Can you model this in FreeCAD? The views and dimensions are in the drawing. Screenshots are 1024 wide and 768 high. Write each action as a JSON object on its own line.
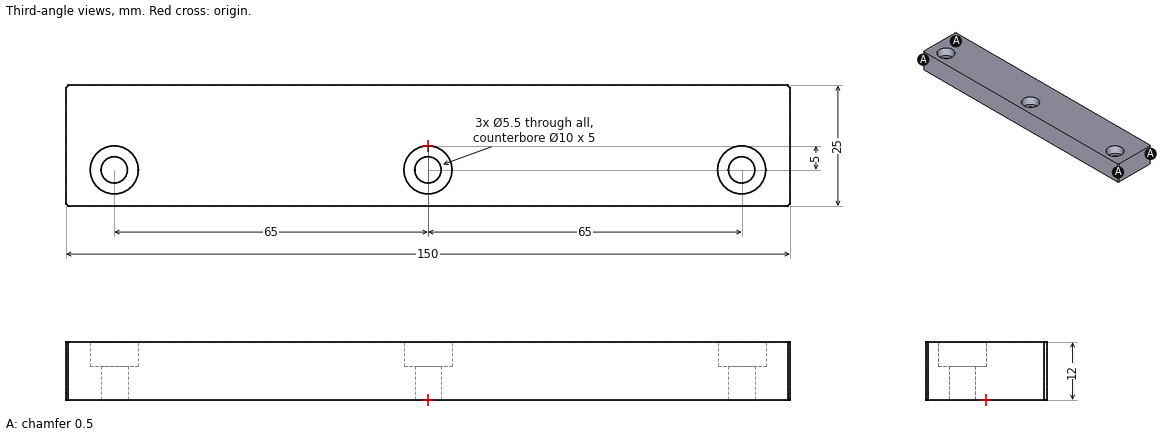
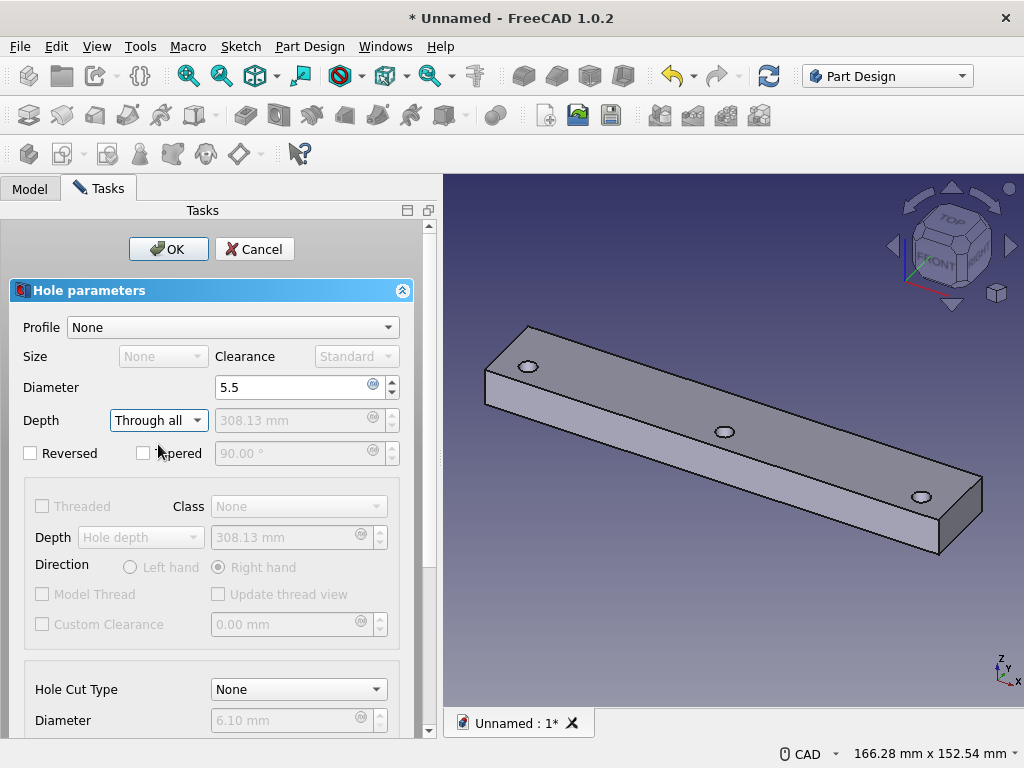
{"action": "left_click", "coordinate": [300, 690]}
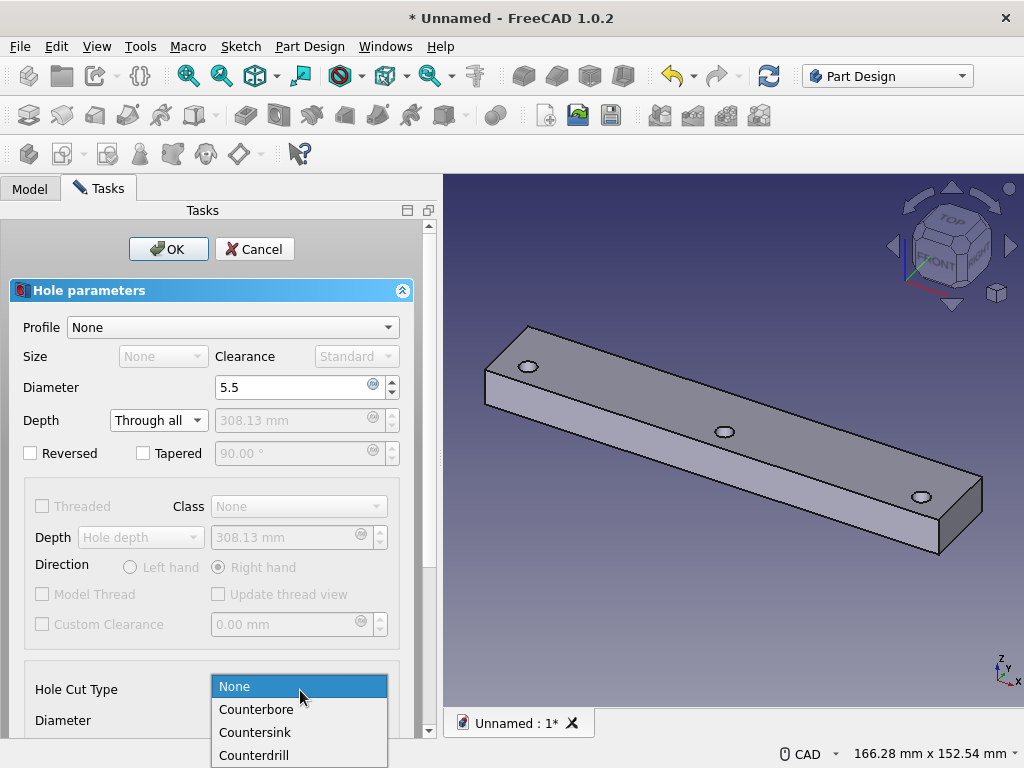
{"action": "left_click", "coordinate": [298, 710]}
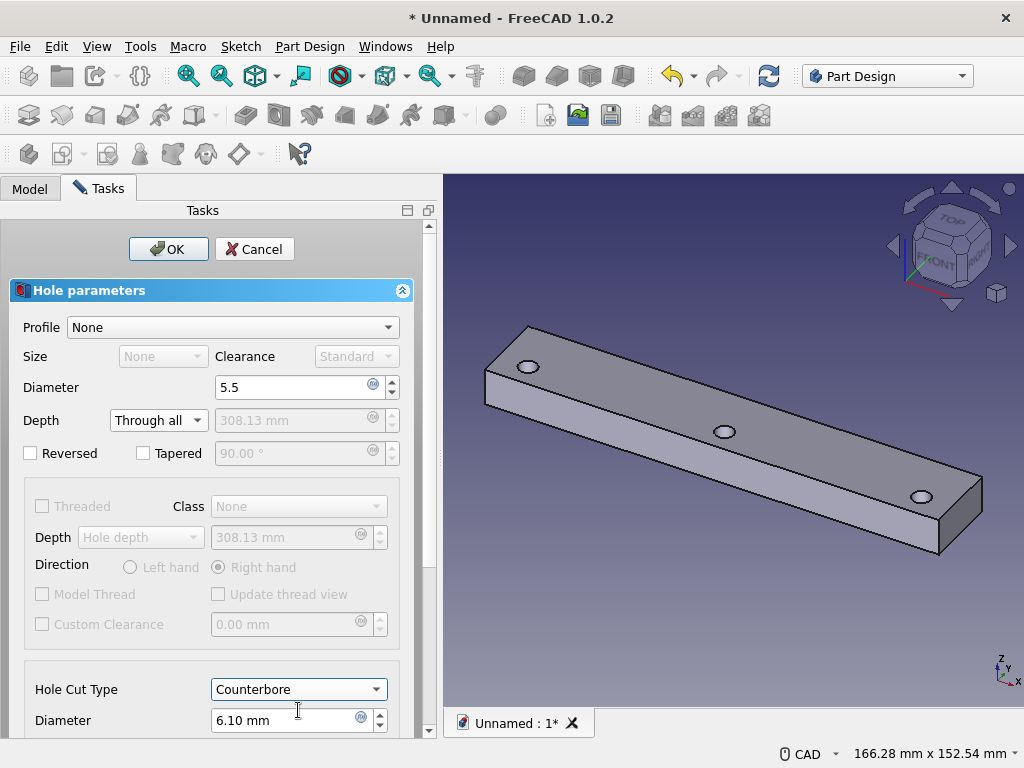
{"action": "triple_click", "coordinate": [292, 720]}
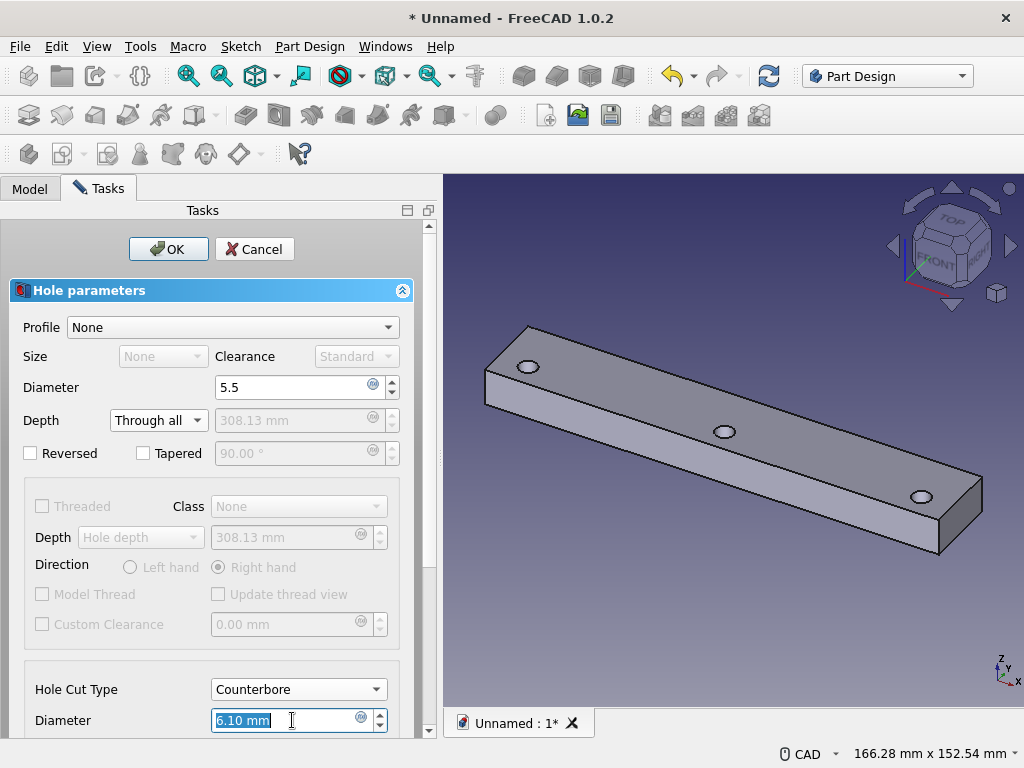
{"action": "type", "text": "10"}
{"action": "key", "text": "Tab"}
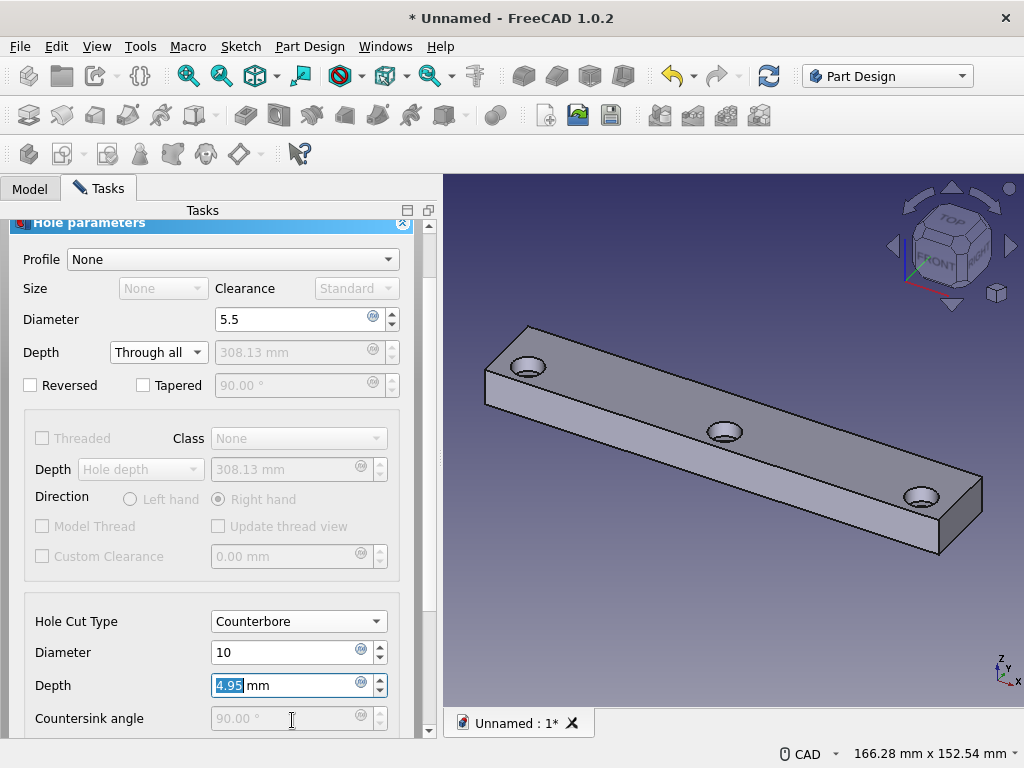
{"action": "type", "text": "5"}
{"action": "key", "text": "Tab"}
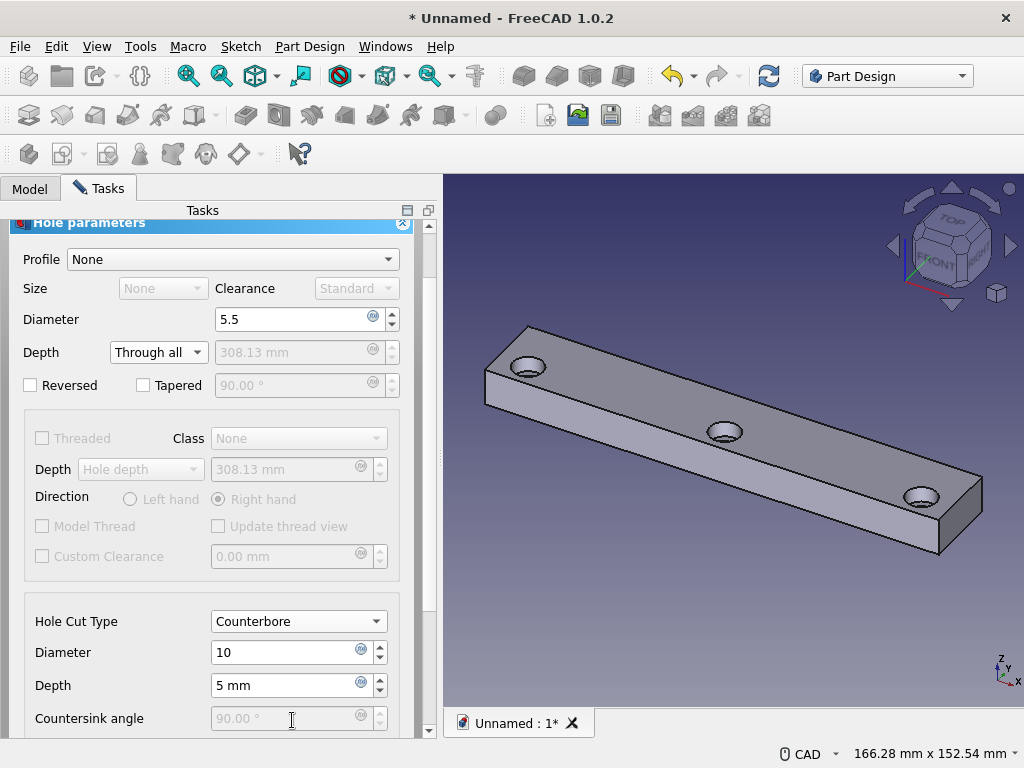
{"action": "scroll", "coordinate": [429, 479], "scroll_direction": "up", "scroll_amount": 2}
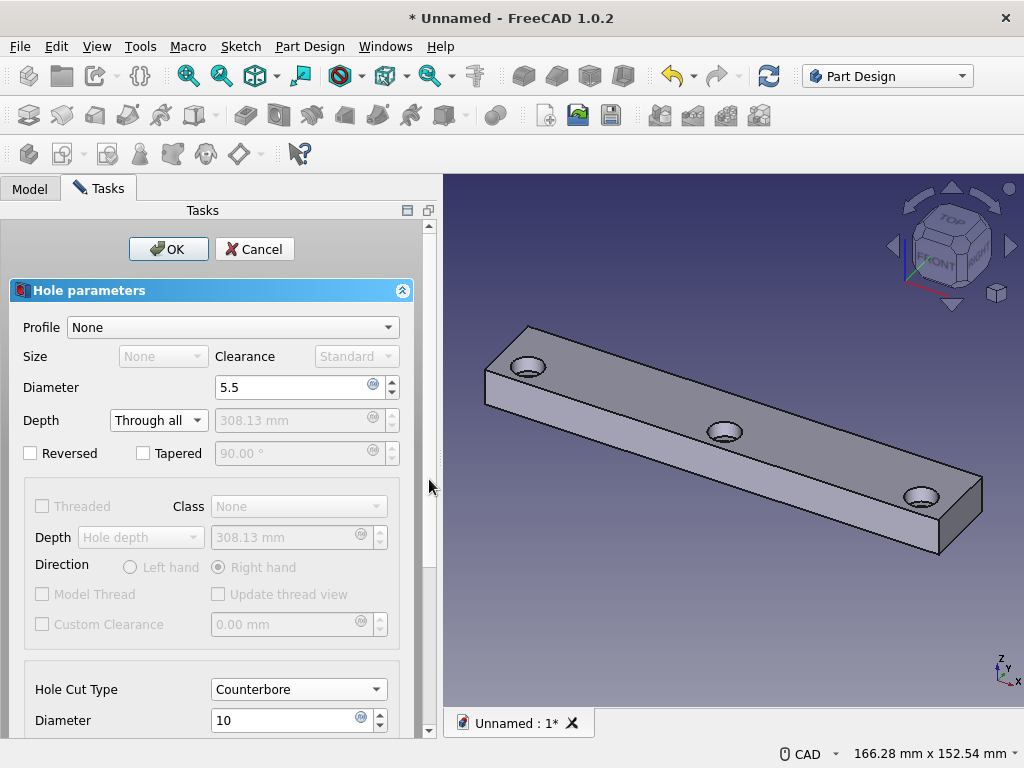
{"action": "left_click", "coordinate": [169, 249]}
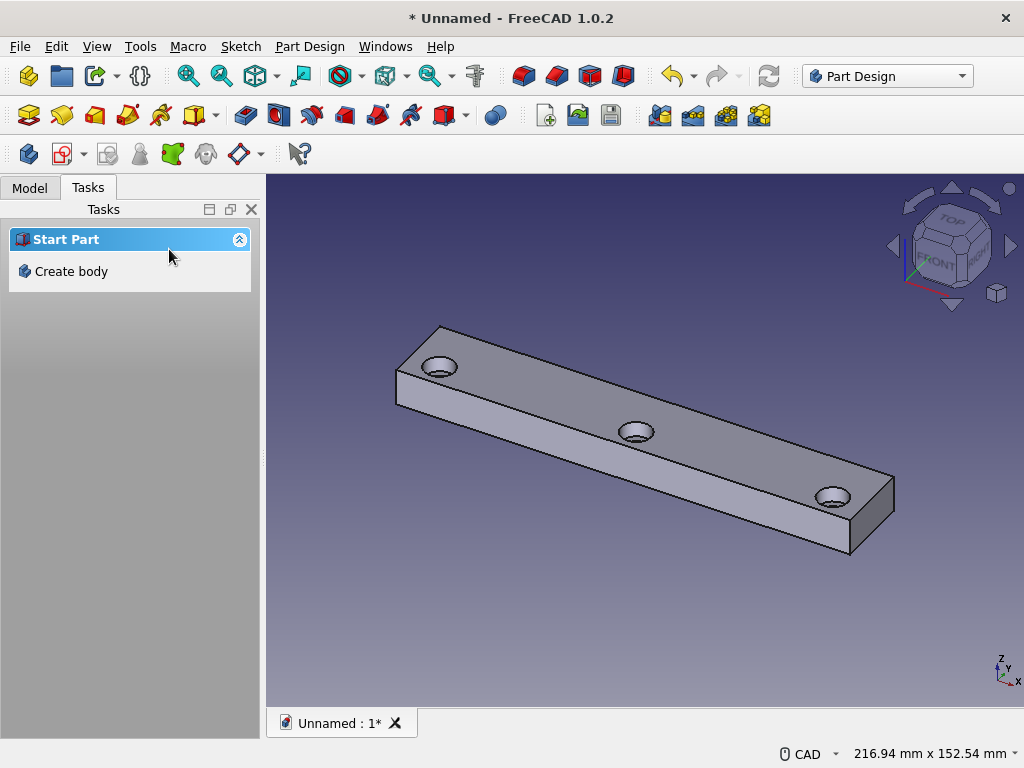
{"action": "left_click", "coordinate": [850, 536]}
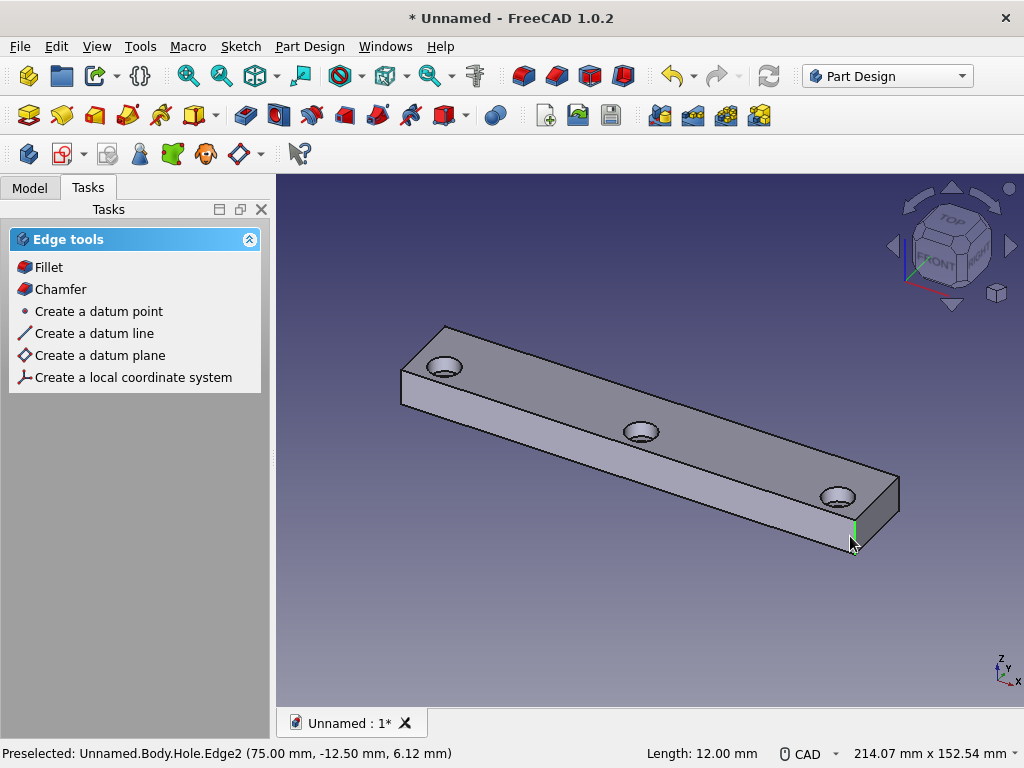
{"action": "key", "text": "0"}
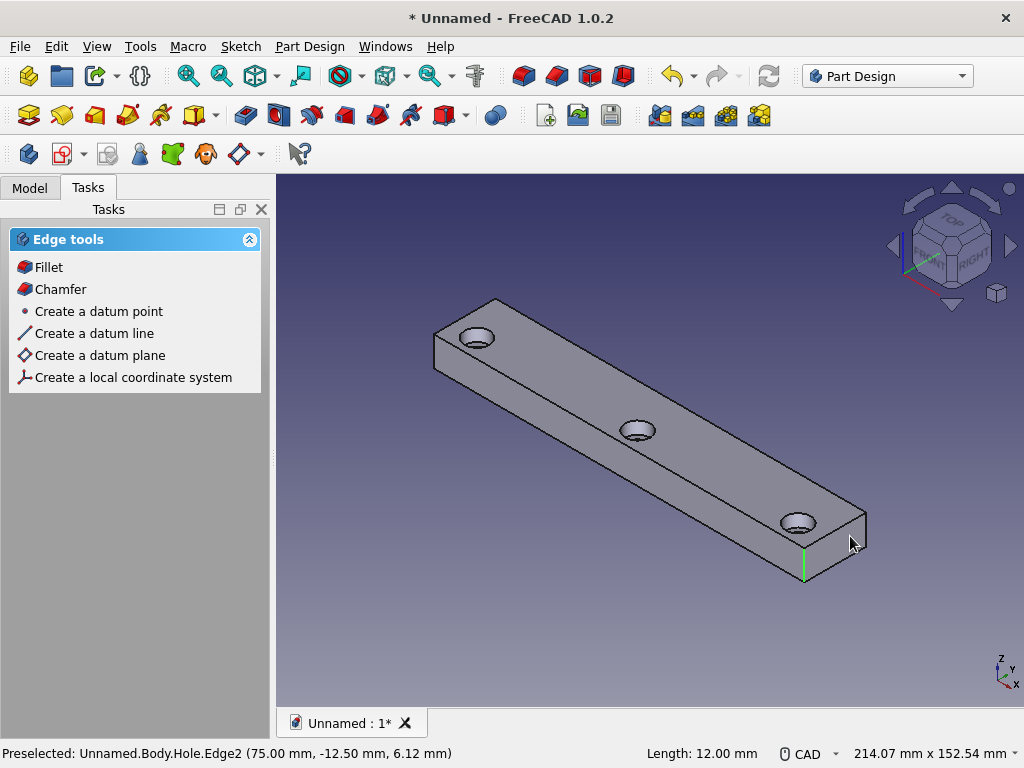
{"action": "key", "text": "2"}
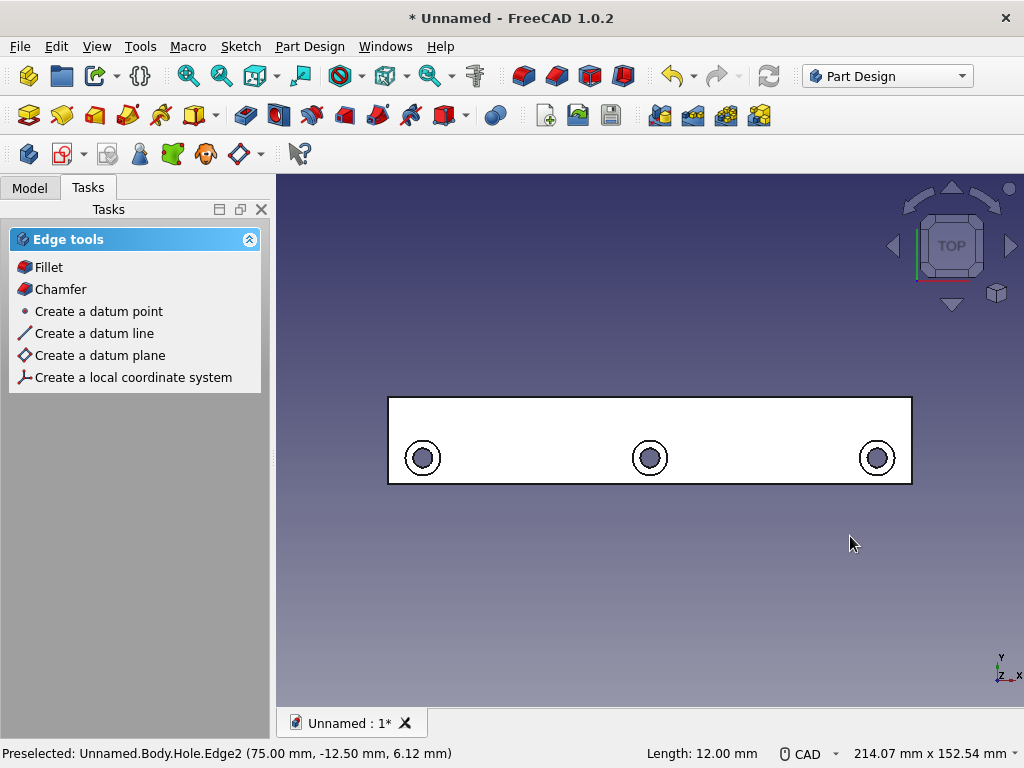
{"action": "key", "text": "1"}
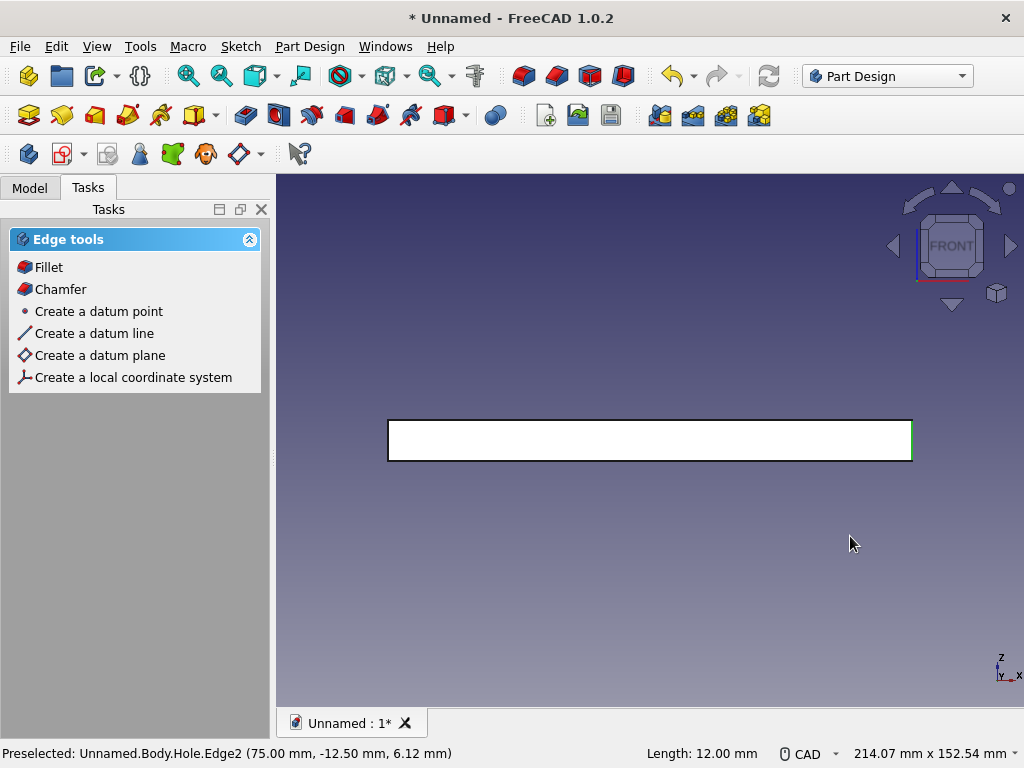
{"action": "left_click", "coordinate": [388, 439], "text": "ctrl"}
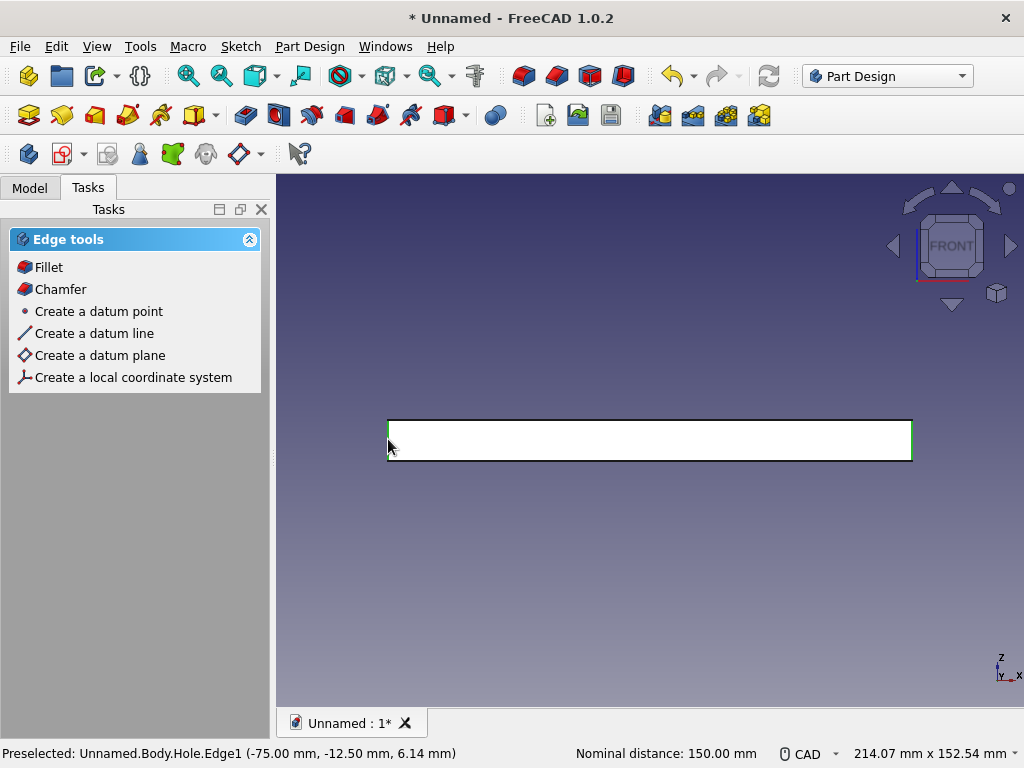
{"action": "key", "text": "3"}